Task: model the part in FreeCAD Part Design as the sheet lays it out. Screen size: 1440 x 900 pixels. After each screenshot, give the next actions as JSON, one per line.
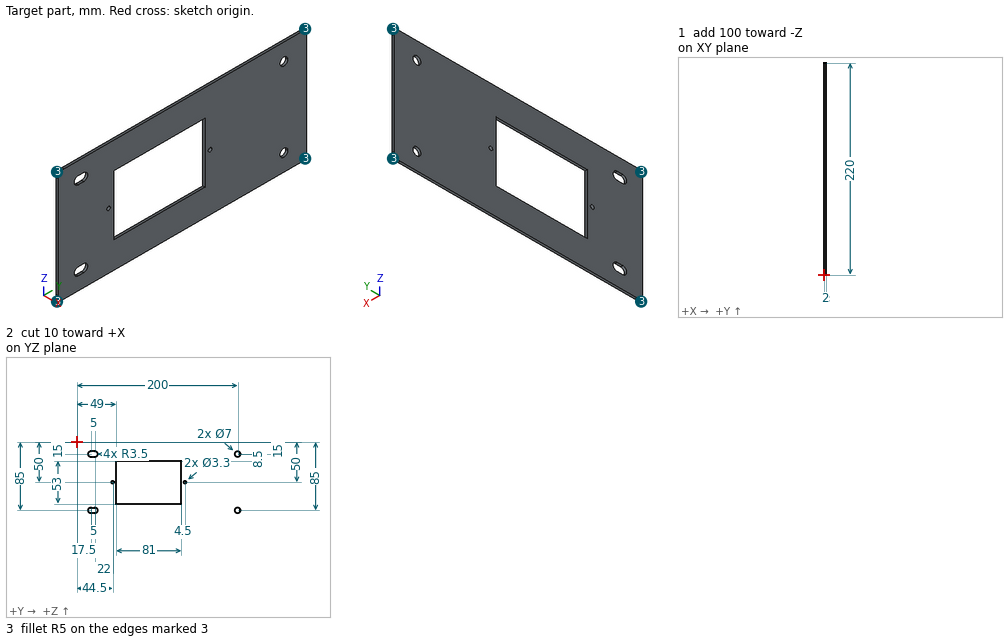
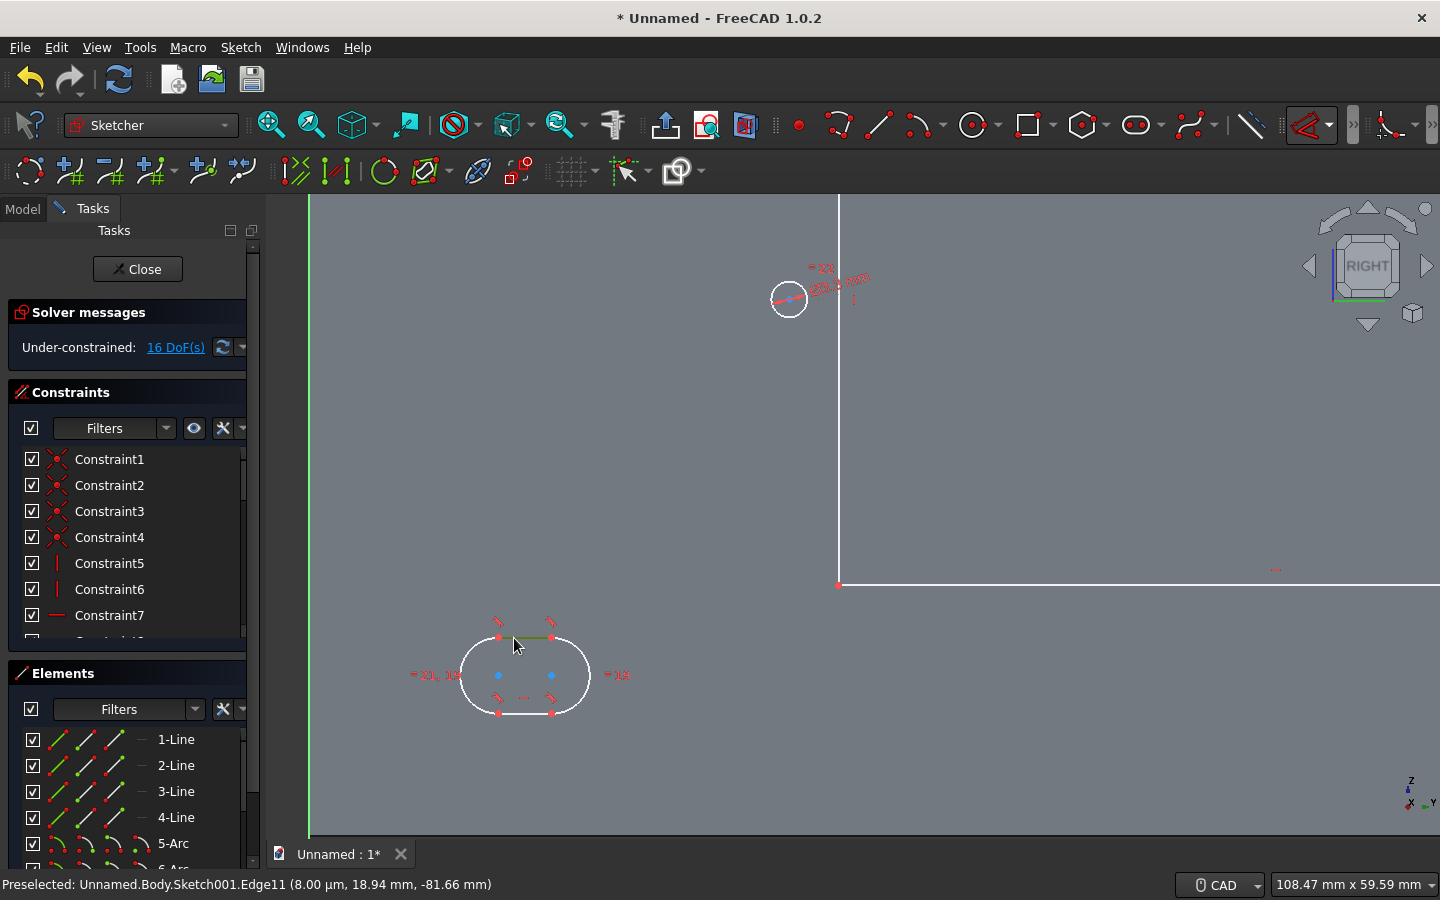
{"action": "left_click", "coordinate": [1332, 126]}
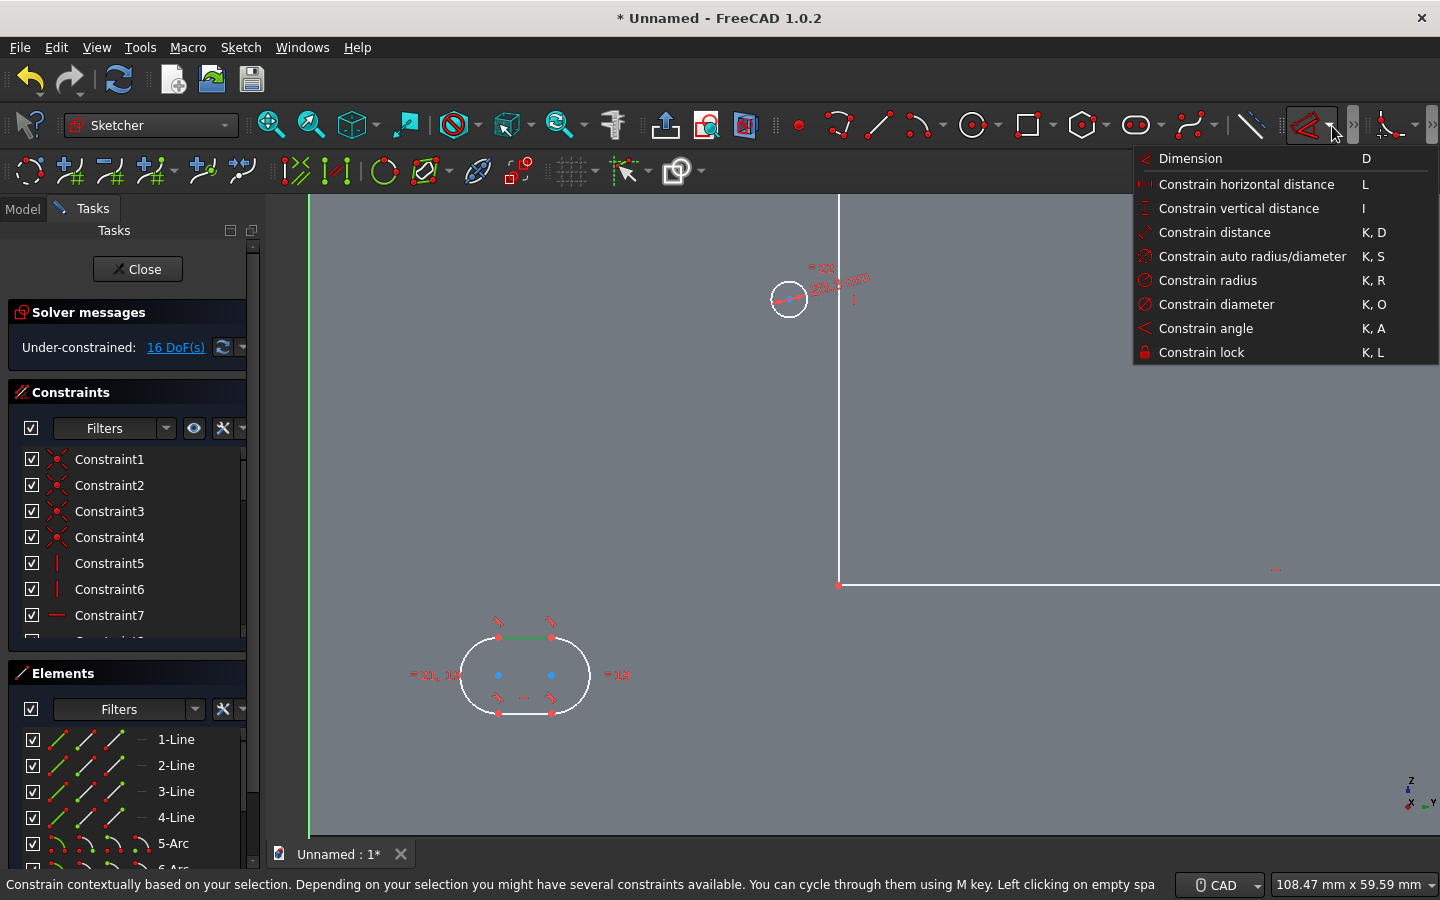
{"action": "left_click", "coordinate": [1286, 184]}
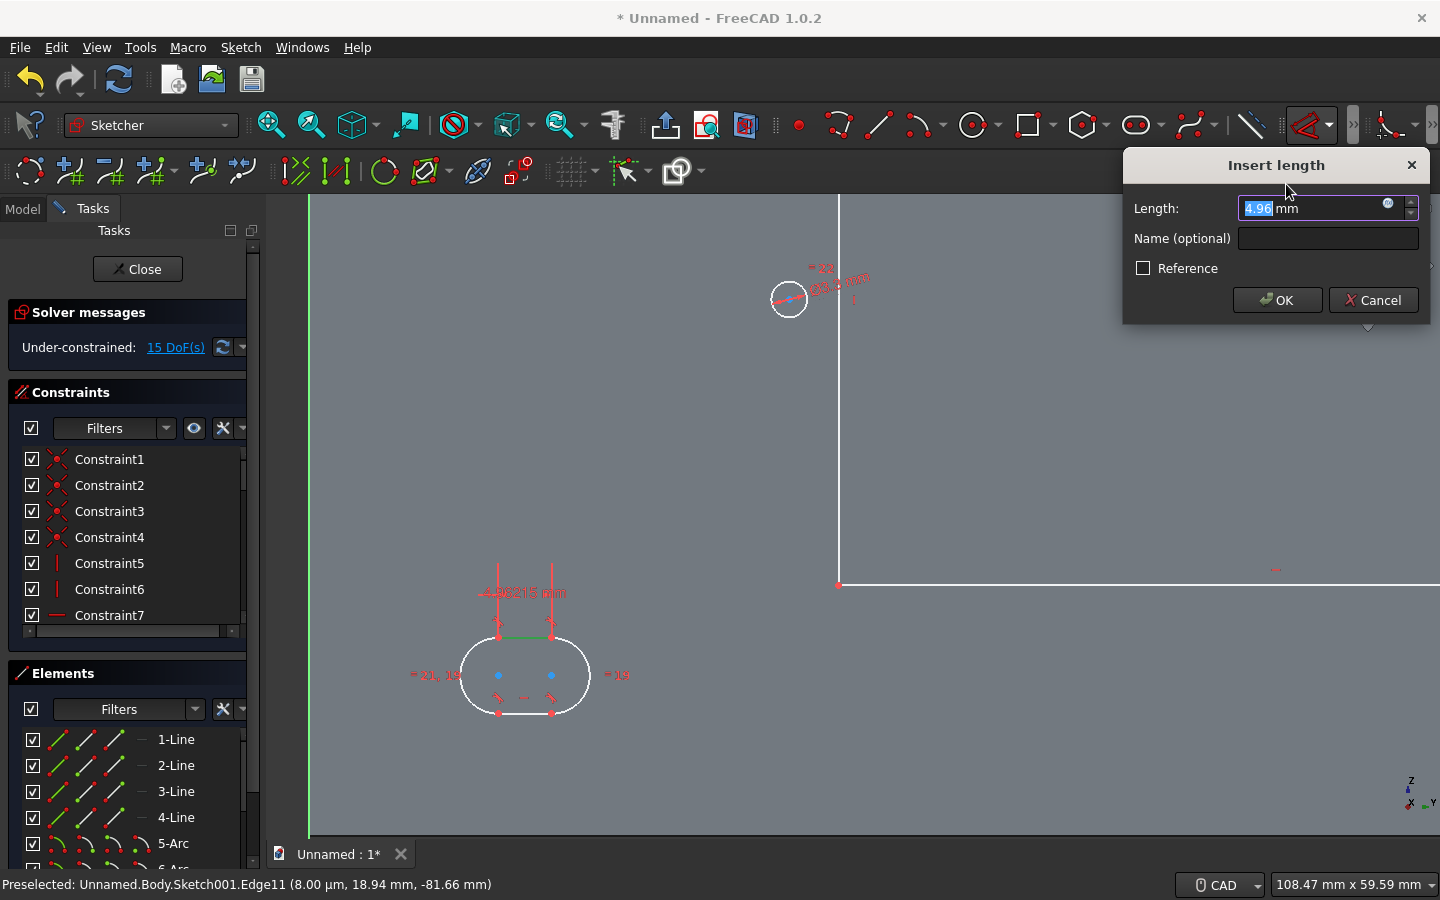
{"action": "type", "text": "5"}
{"action": "key", "text": "Return"}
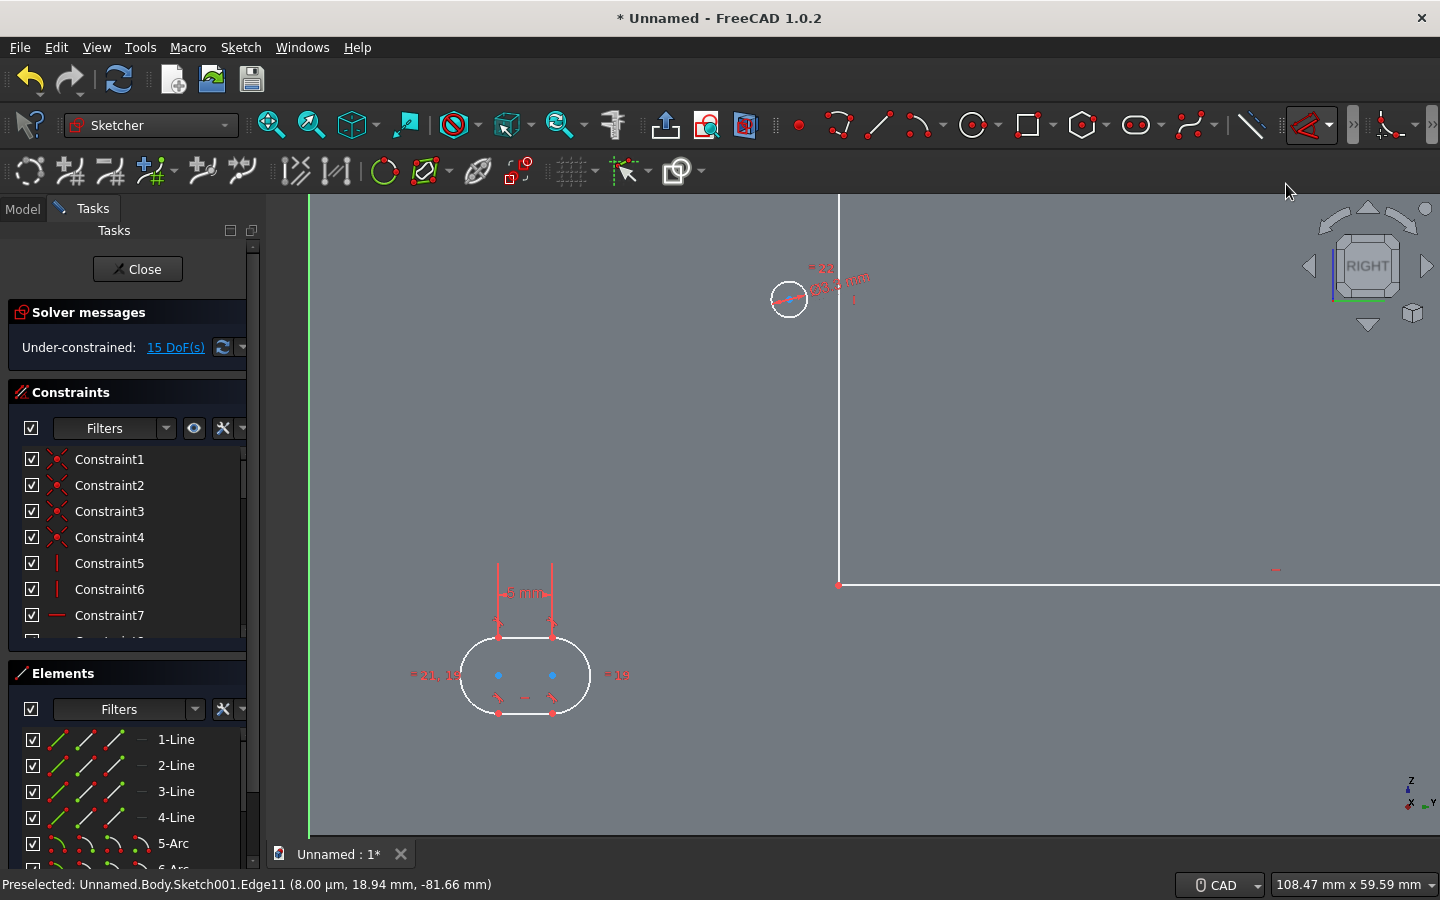
{"action": "scroll", "coordinate": [515, 639], "scroll_direction": "down", "scroll_amount": 6}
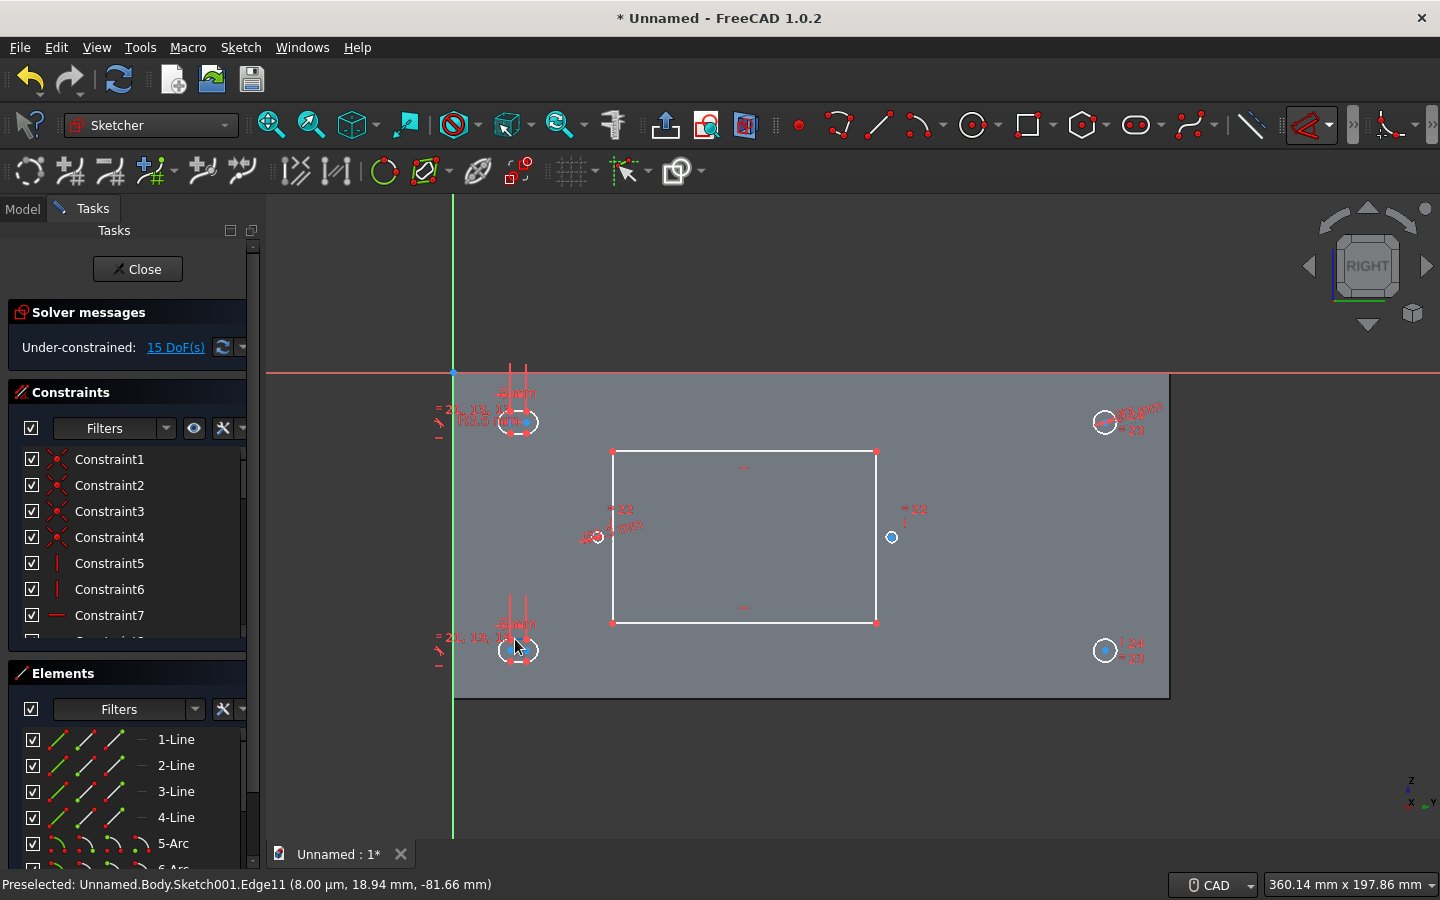
{"action": "left_click", "coordinate": [613, 572]}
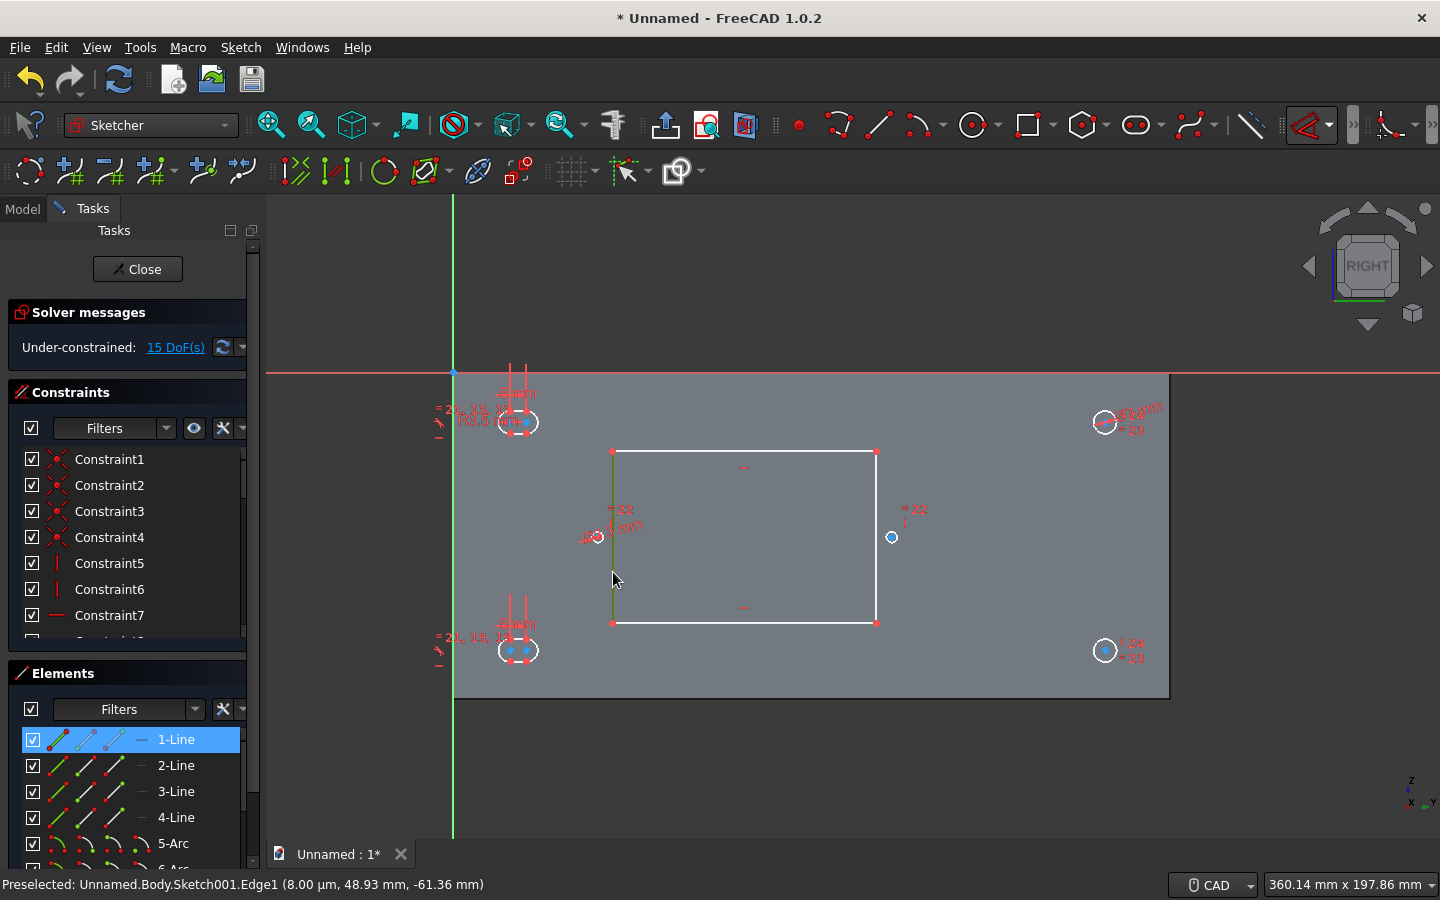
{"action": "left_click", "coordinate": [1332, 126]}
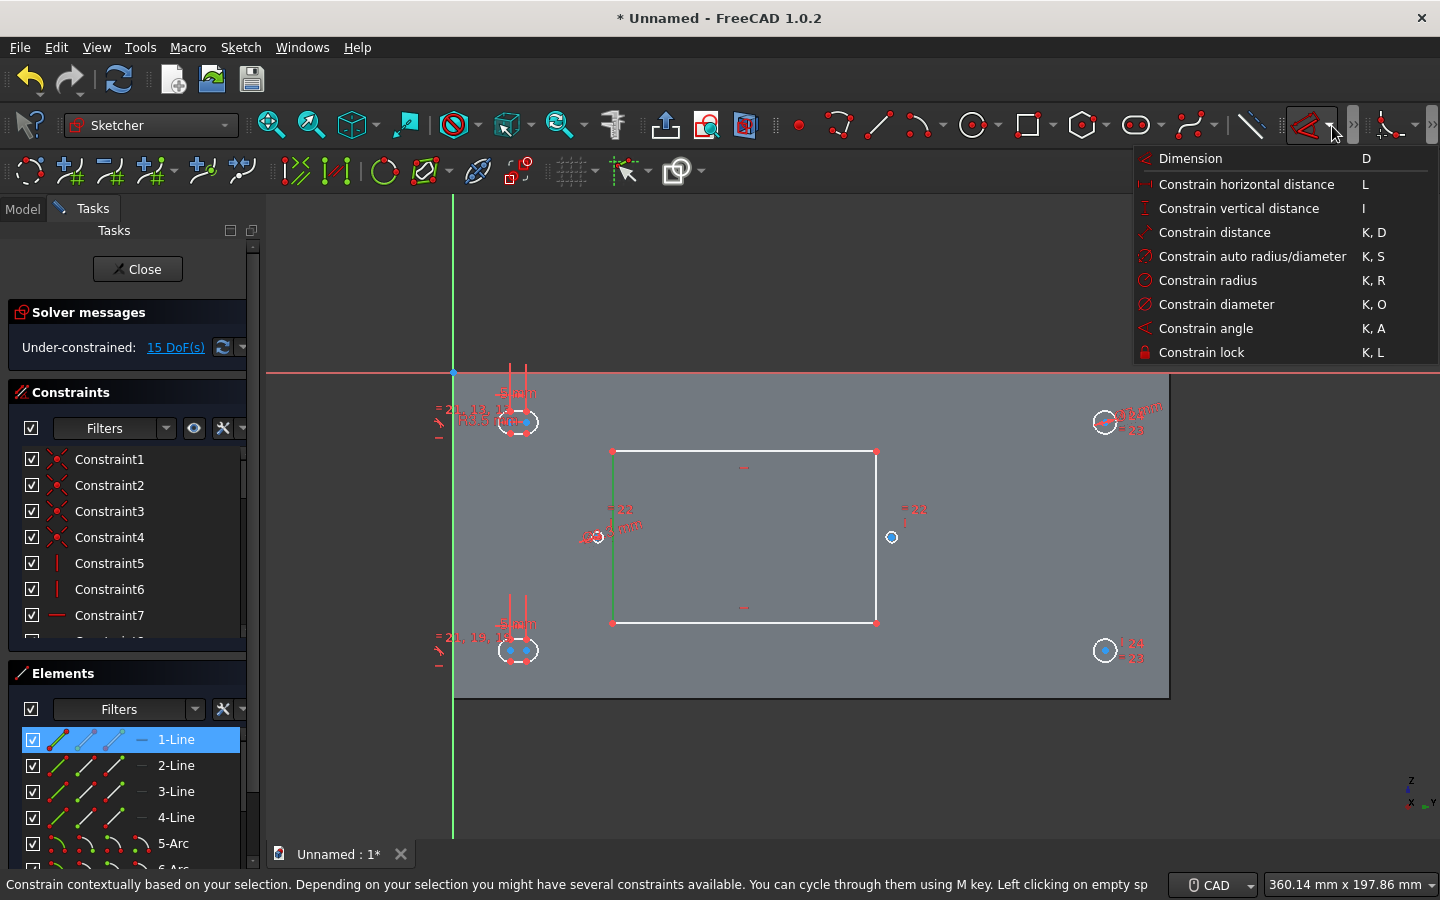
{"action": "left_click", "coordinate": [1286, 208]}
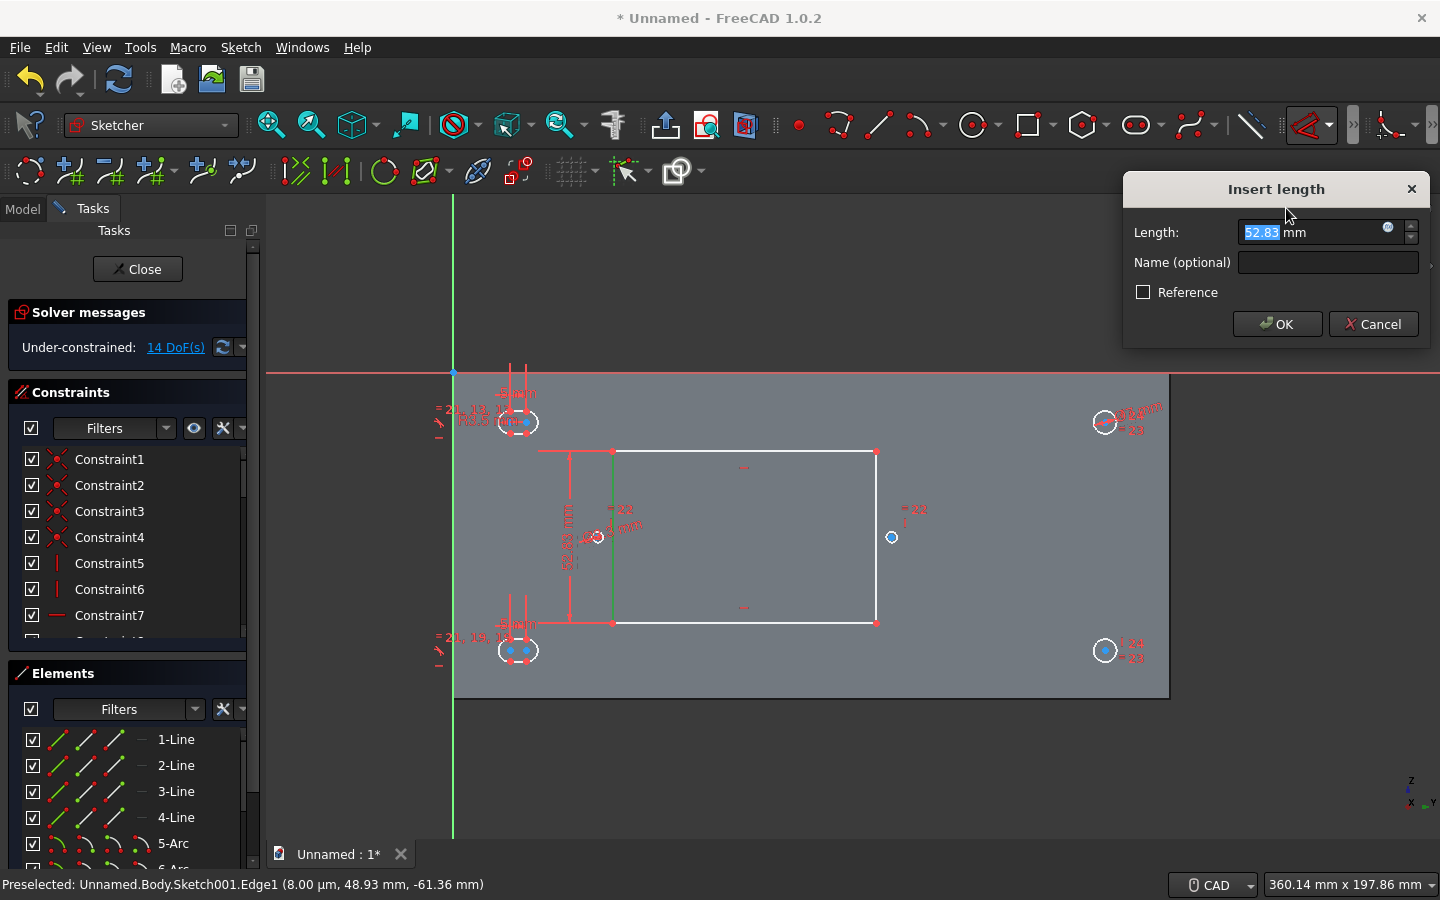
{"action": "type", "text": "53"}
{"action": "key", "text": "Return"}